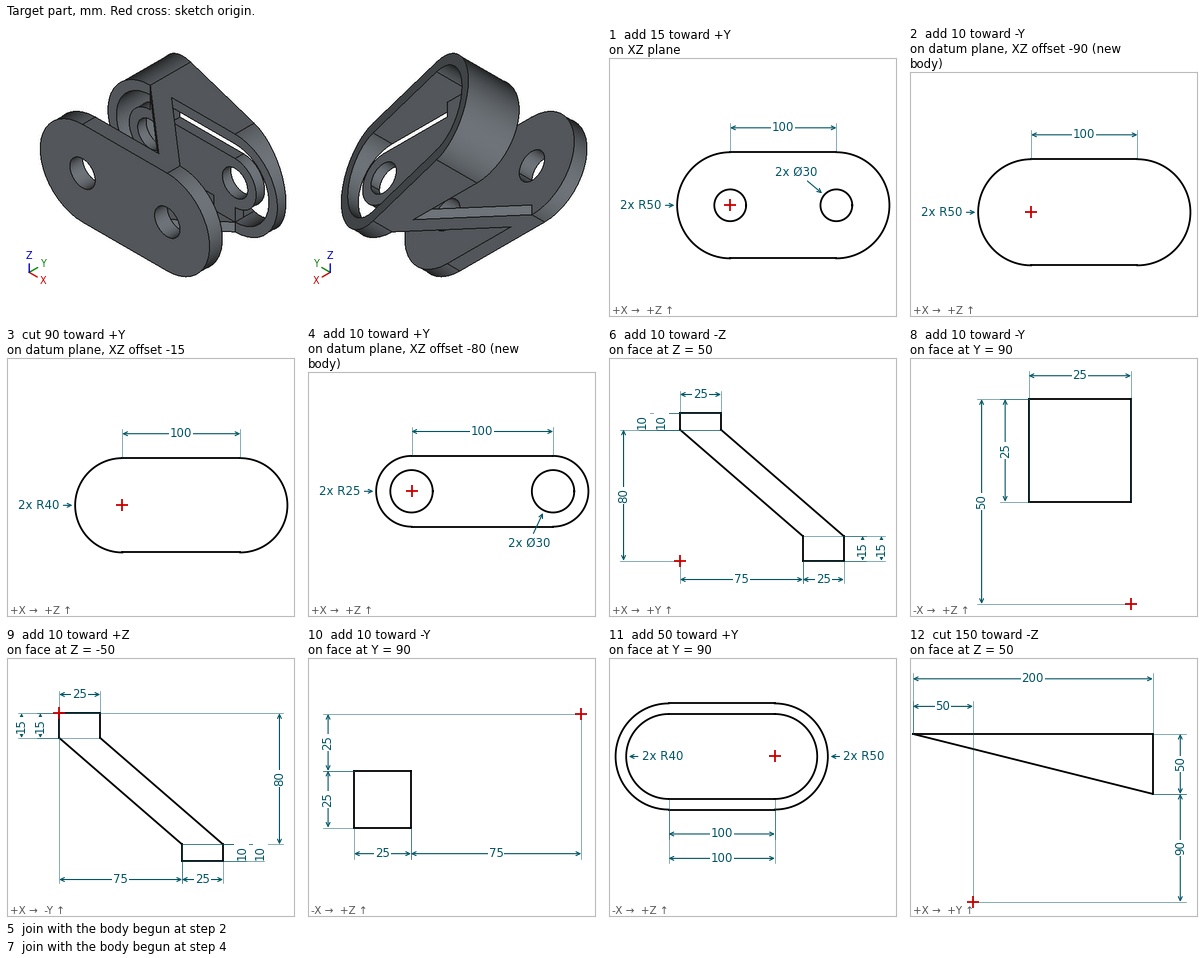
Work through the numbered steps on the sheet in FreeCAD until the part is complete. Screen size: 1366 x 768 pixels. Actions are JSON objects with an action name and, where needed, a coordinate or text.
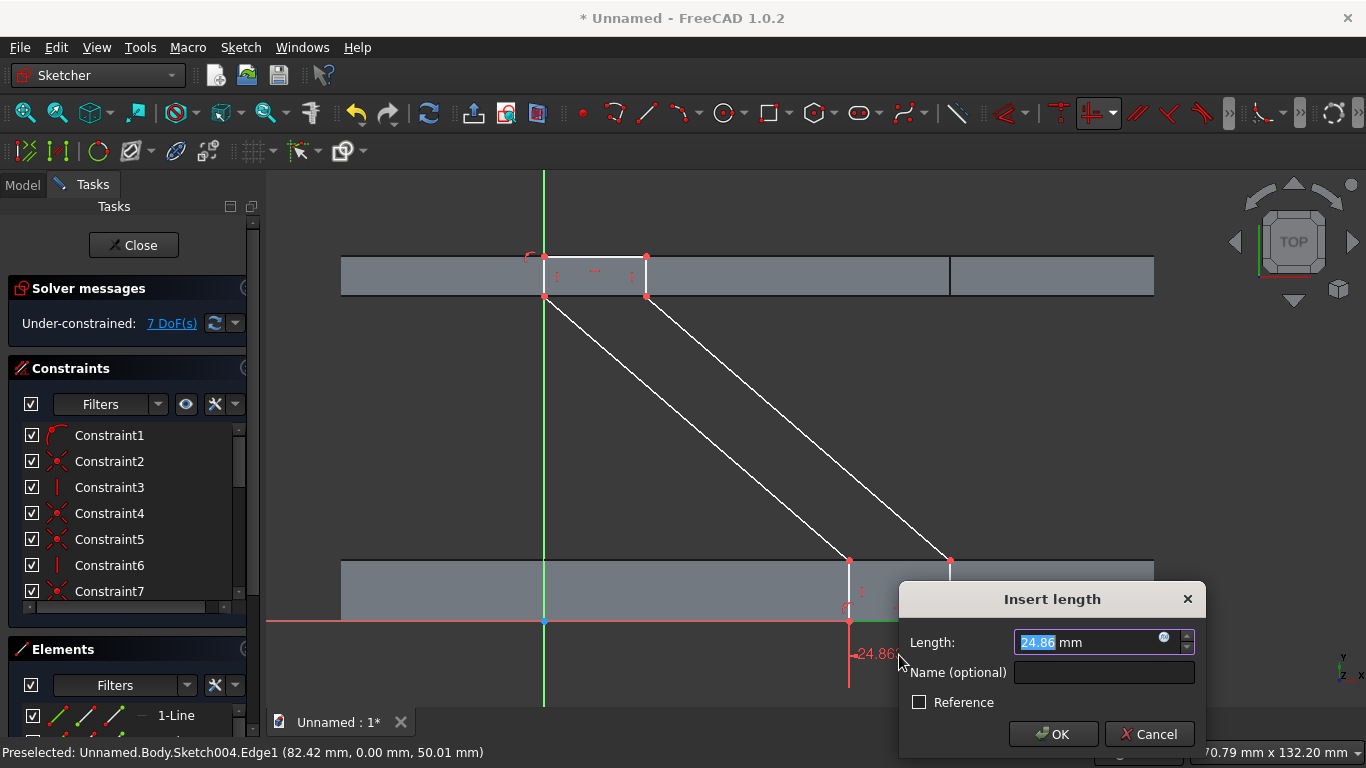
{"action": "type", "text": "25"}
{"action": "key", "text": "Return"}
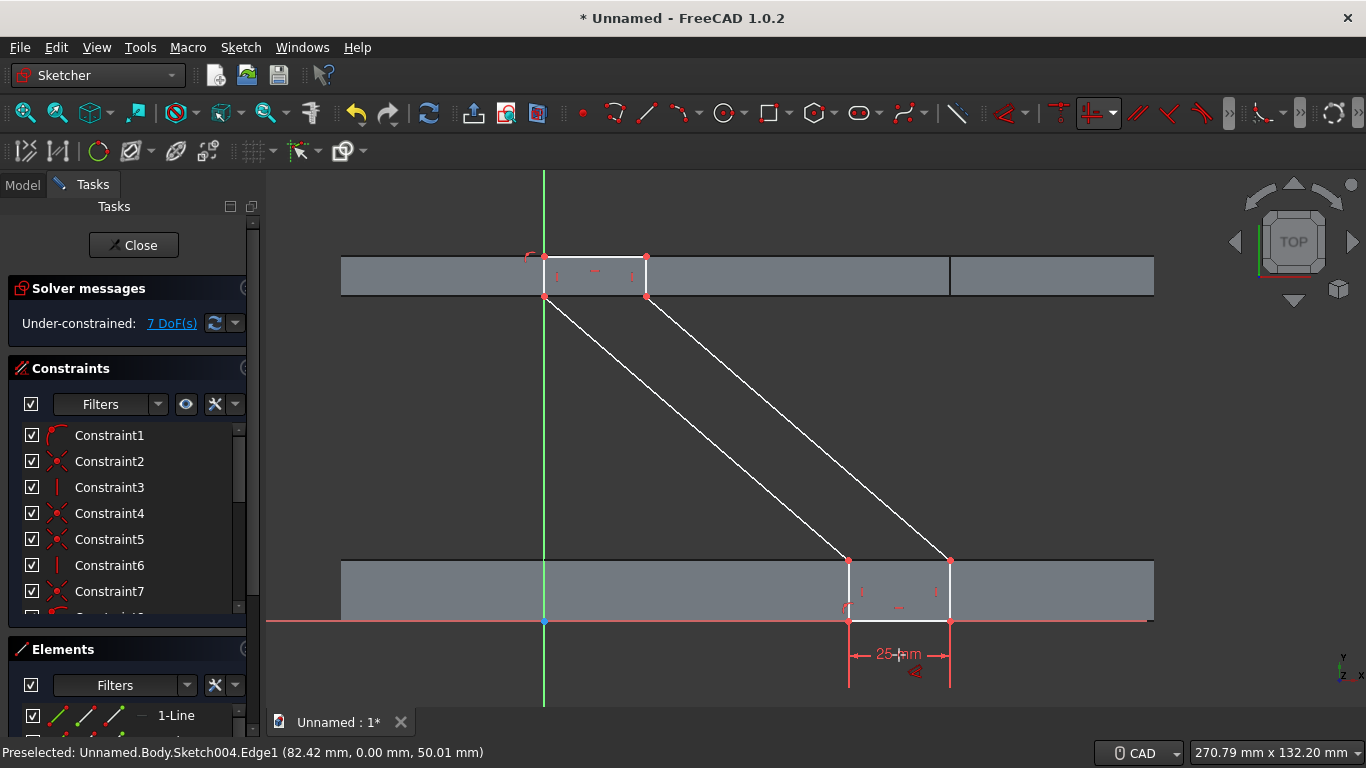
{"action": "left_click", "coordinate": [950, 603]}
{"action": "left_click", "coordinate": [984, 591]}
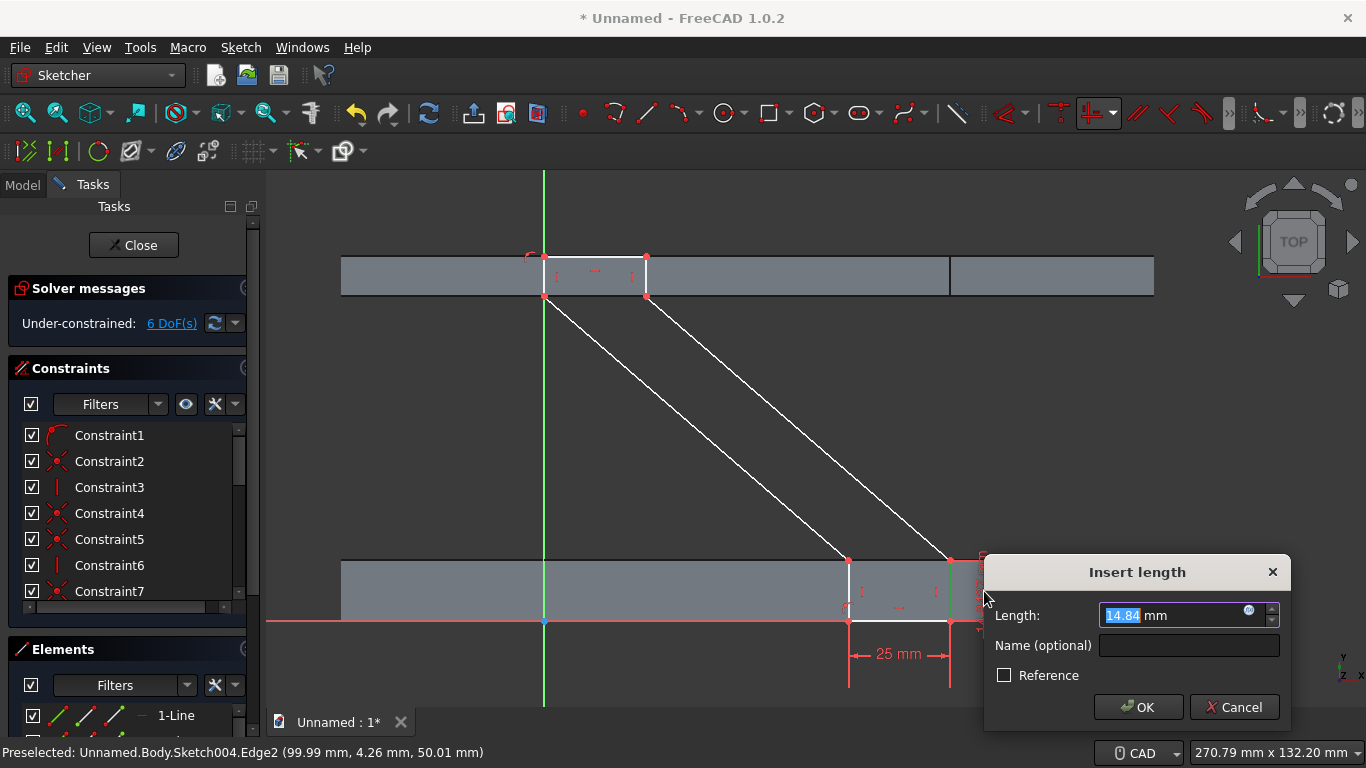
{"action": "type", "text": "15"}
{"action": "key", "text": "Return"}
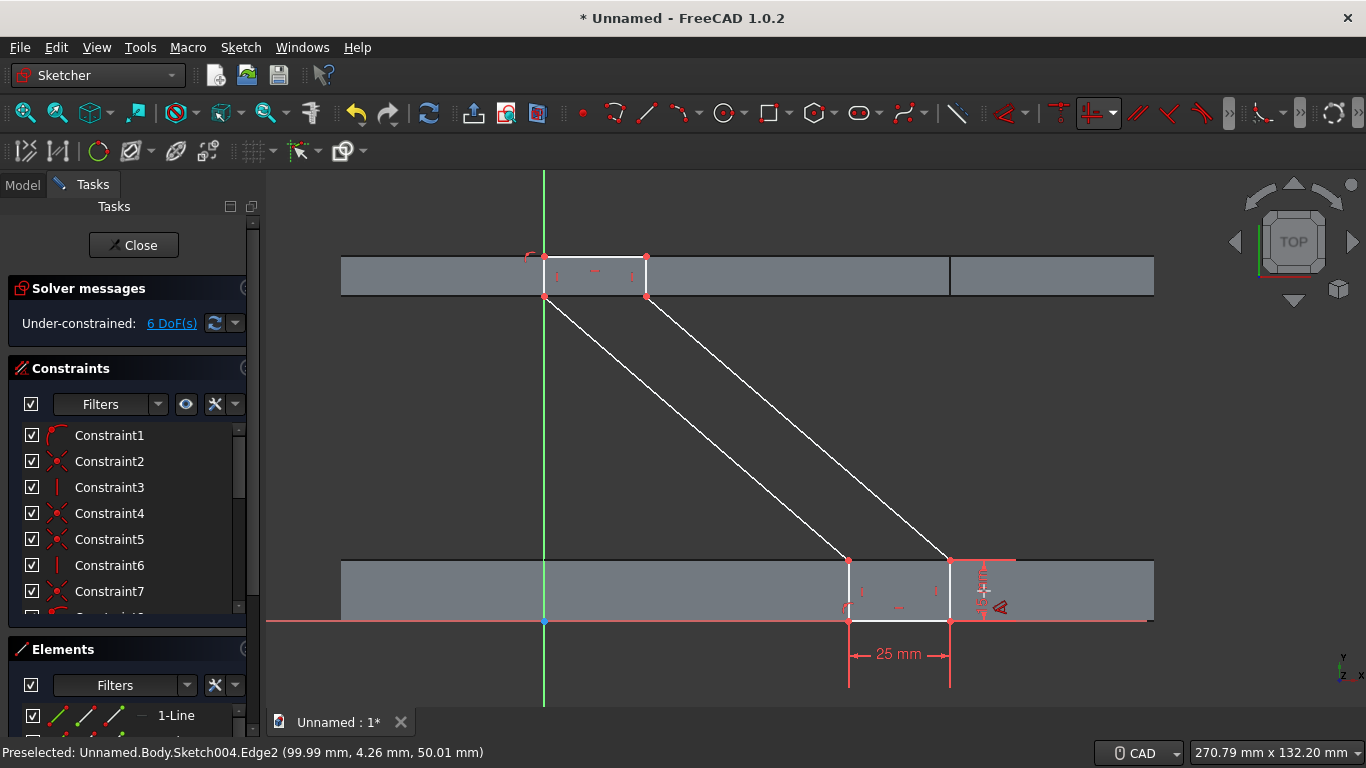
{"action": "left_click", "coordinate": [646, 285]}
{"action": "left_click", "coordinate": [612, 277]}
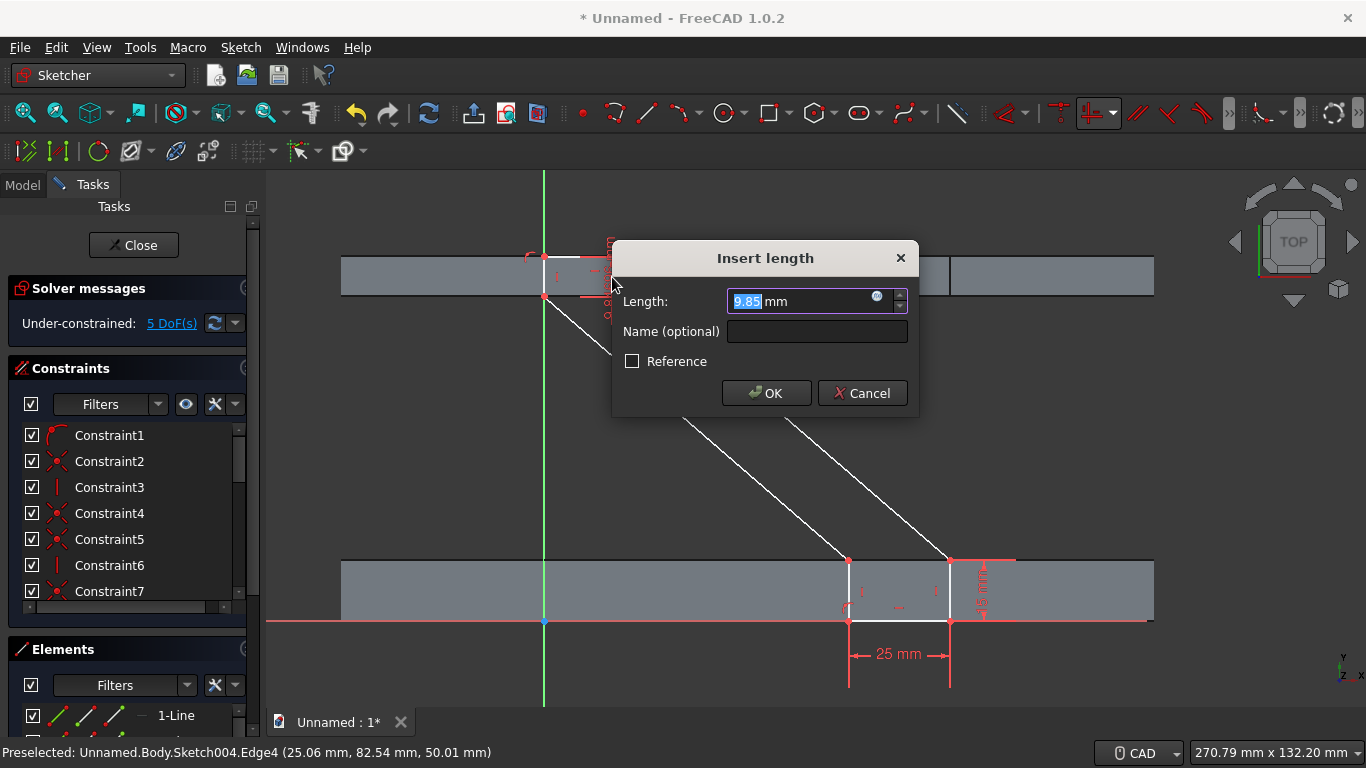
{"action": "type", "text": "10"}
{"action": "key", "text": "Return"}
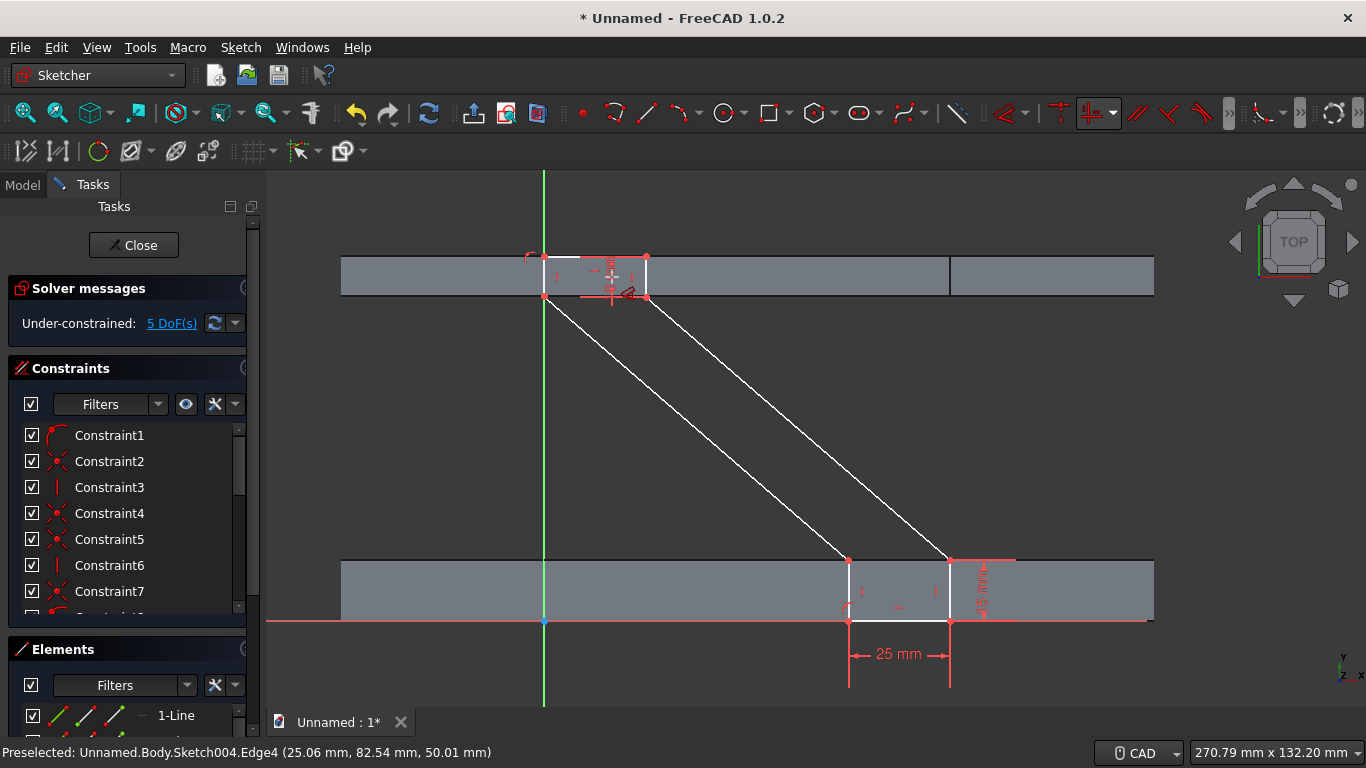
{"action": "left_click", "coordinate": [615, 257]}
{"action": "left_click", "coordinate": [595, 223]}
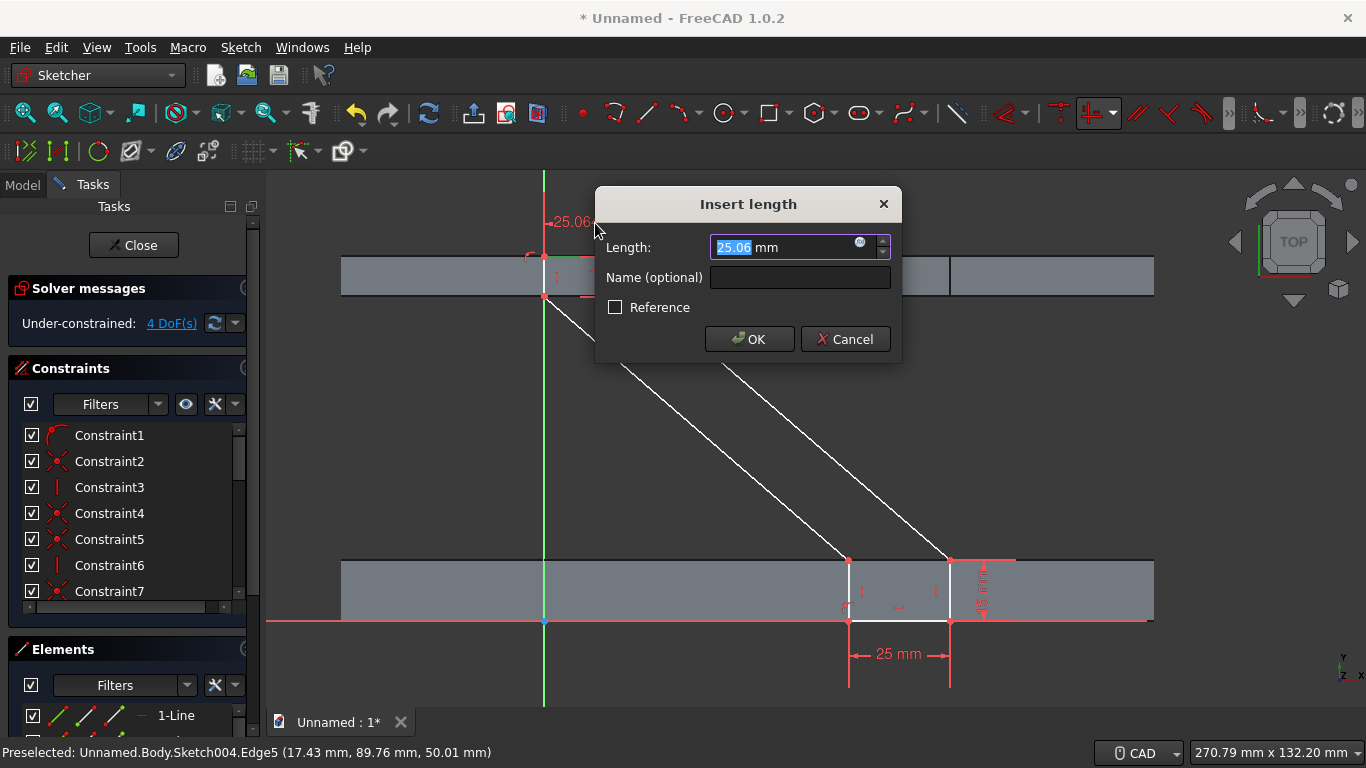
{"action": "type", "text": "25"}
{"action": "key", "text": "Return"}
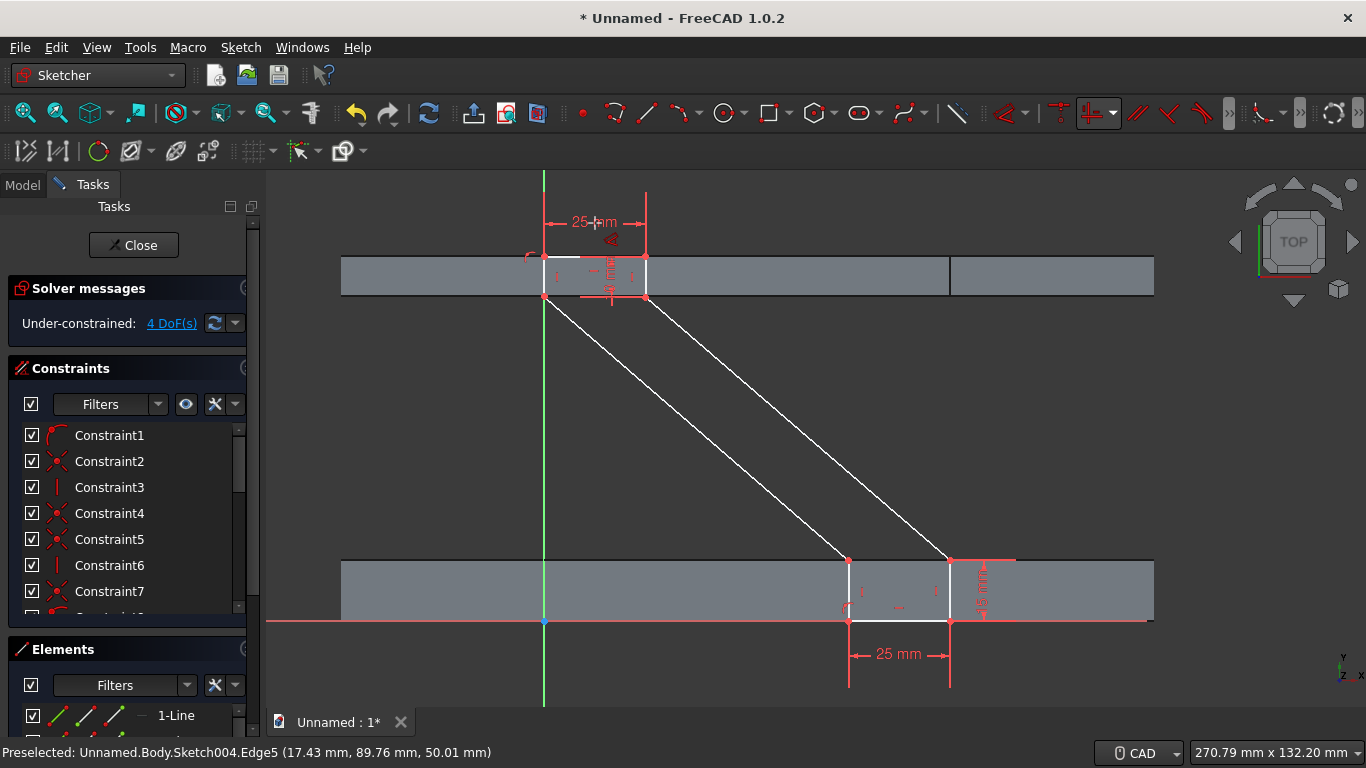
{"action": "left_click", "coordinate": [544, 269]}
{"action": "left_click", "coordinate": [510, 277]}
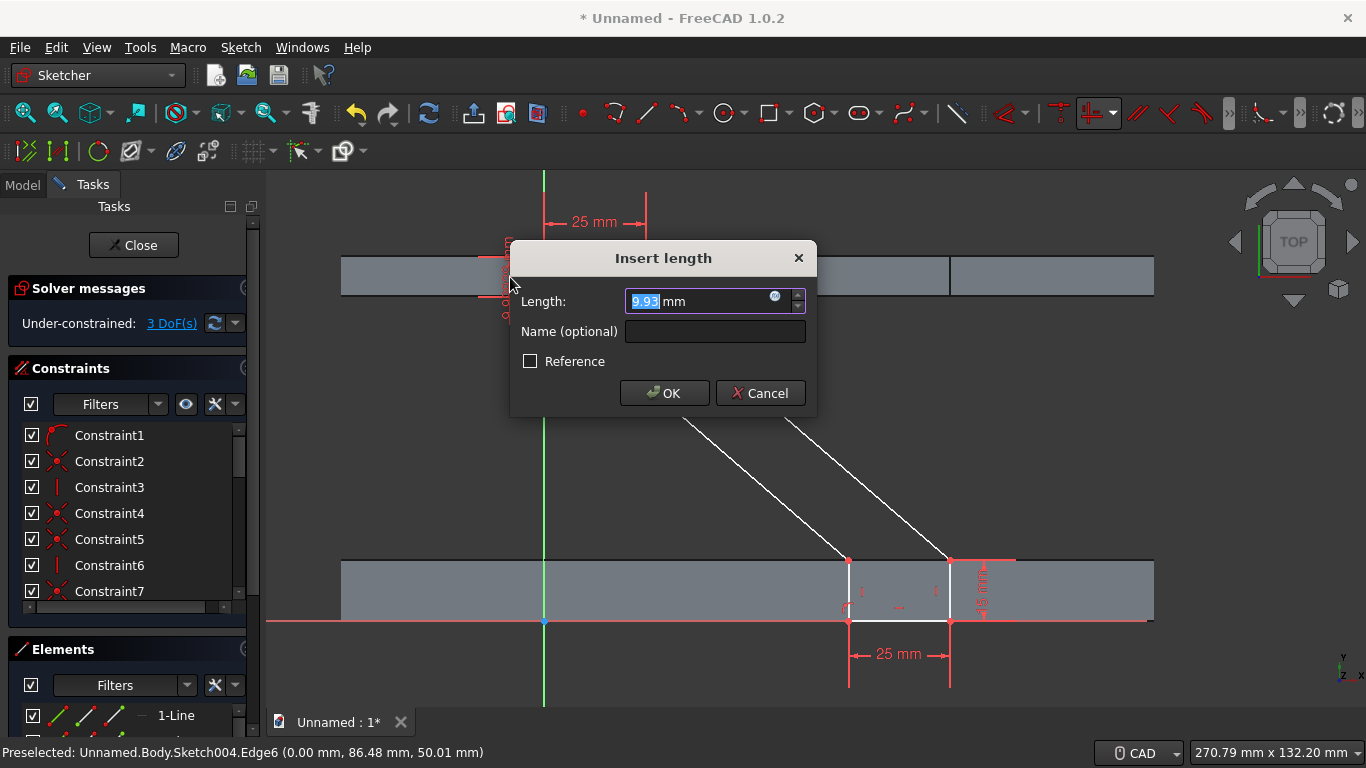
{"action": "type", "text": "10"}
{"action": "key", "text": "Return"}